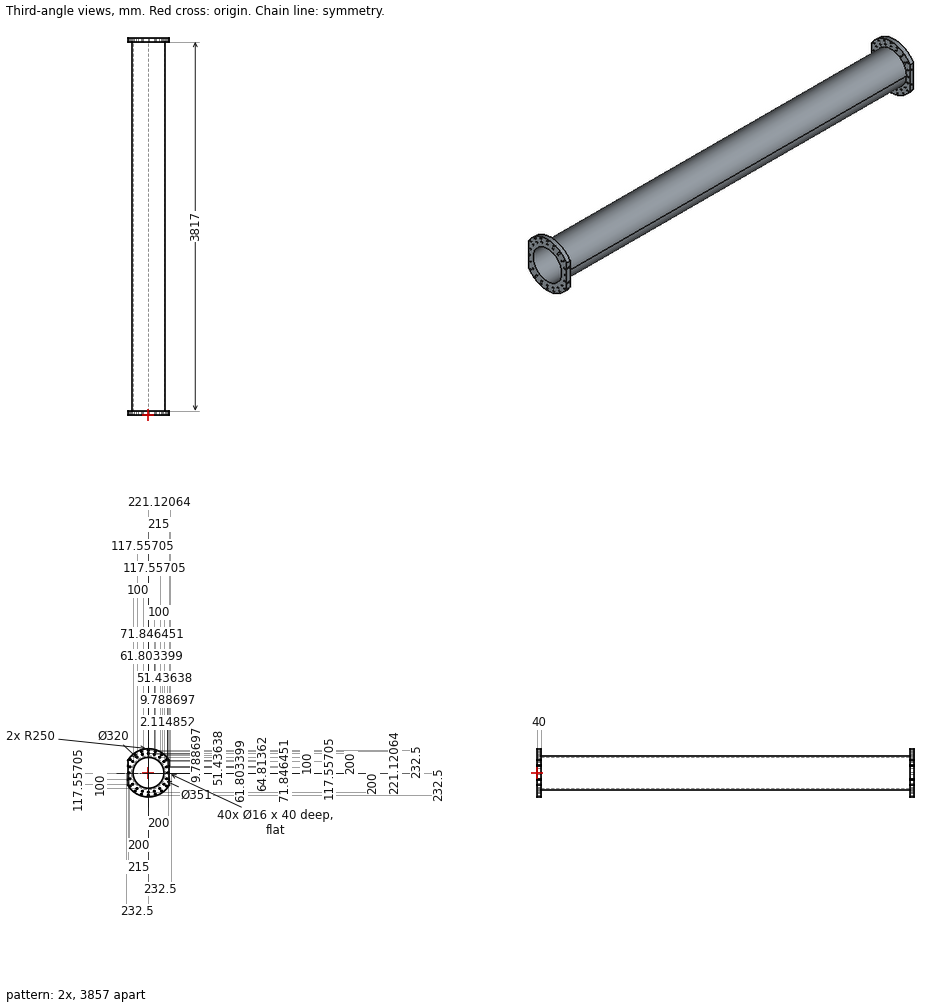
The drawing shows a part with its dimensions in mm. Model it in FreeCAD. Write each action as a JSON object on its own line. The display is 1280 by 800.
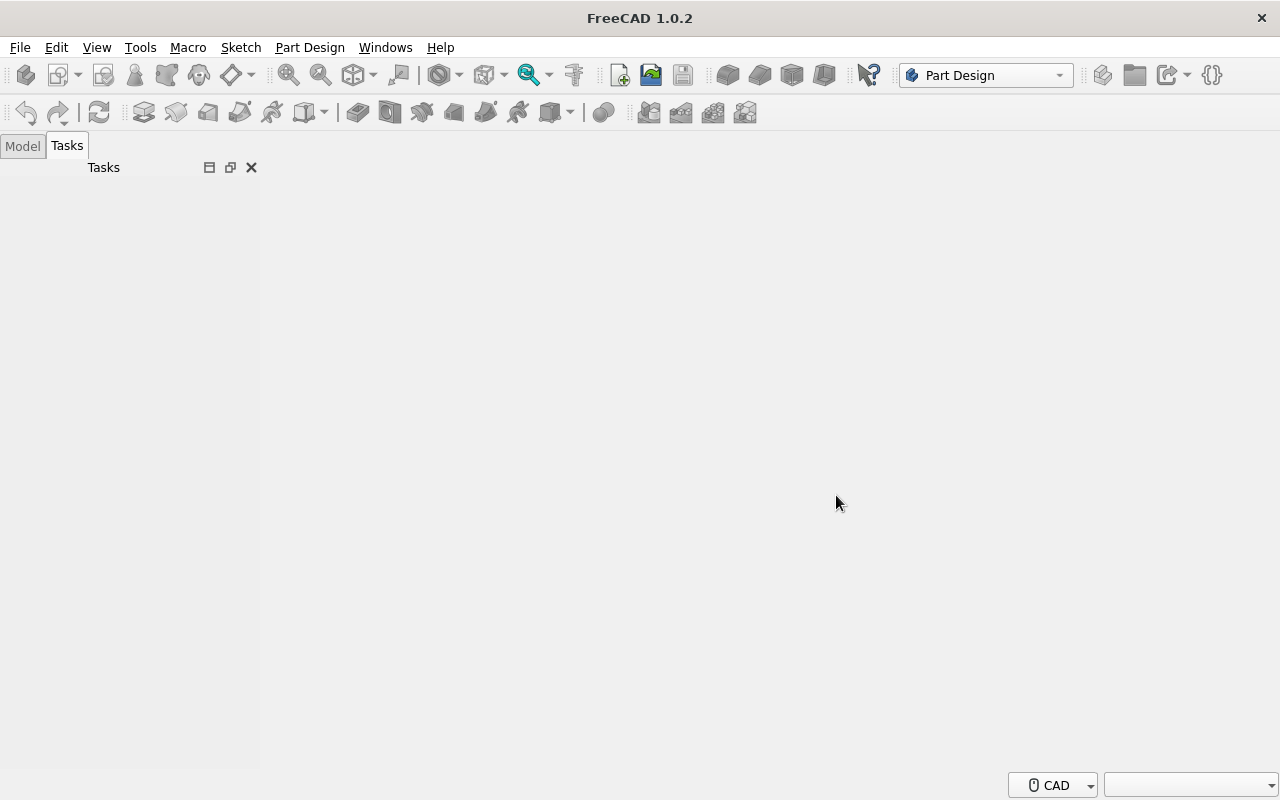
{"action": "left_click", "coordinate": [620, 76]}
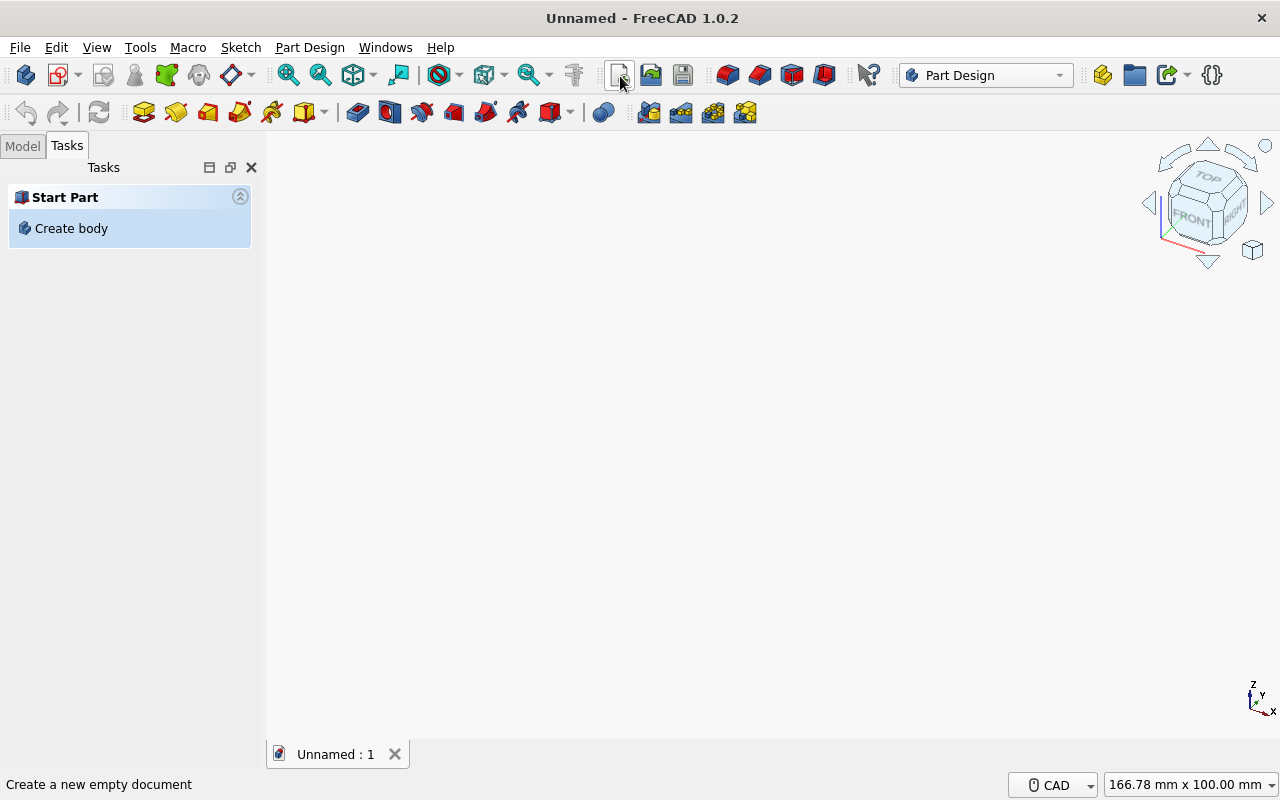
{"action": "left_click", "coordinate": [58, 76]}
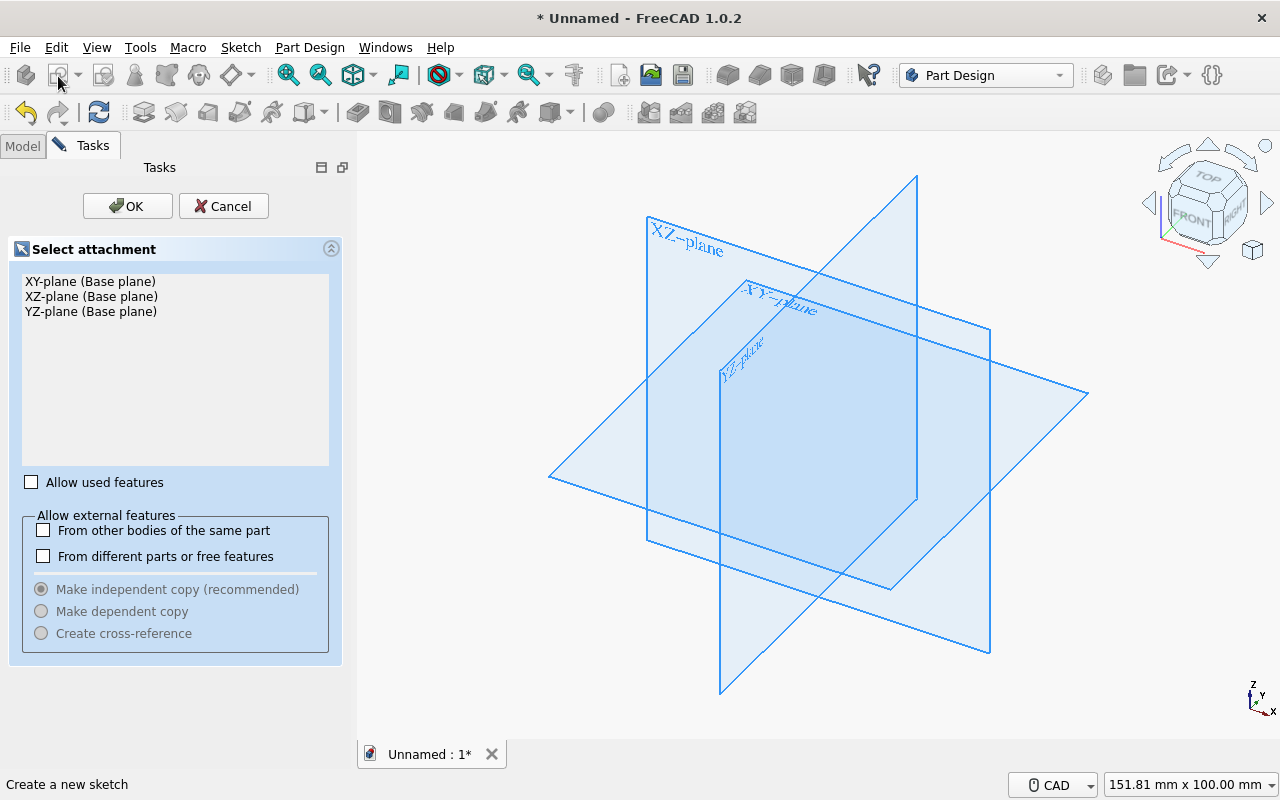
{"action": "left_click", "coordinate": [82, 296]}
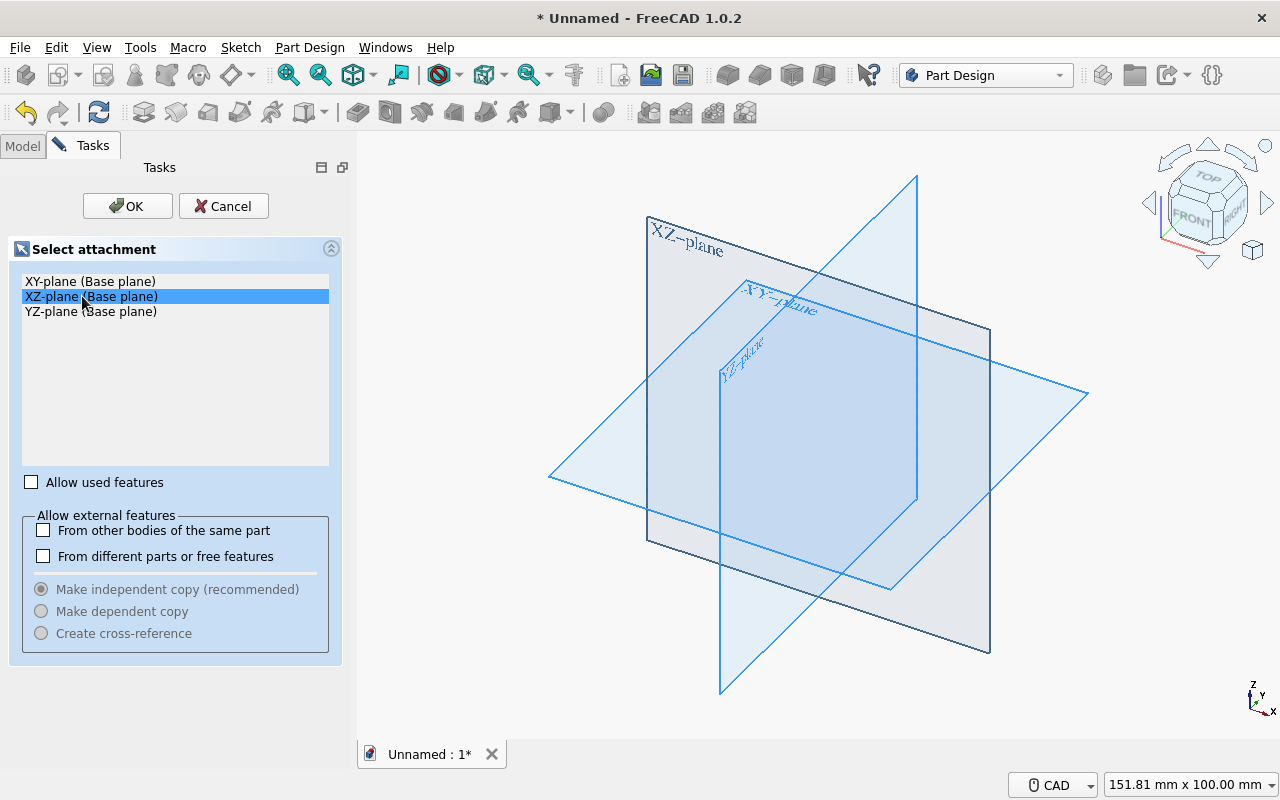
{"action": "left_click", "coordinate": [128, 206]}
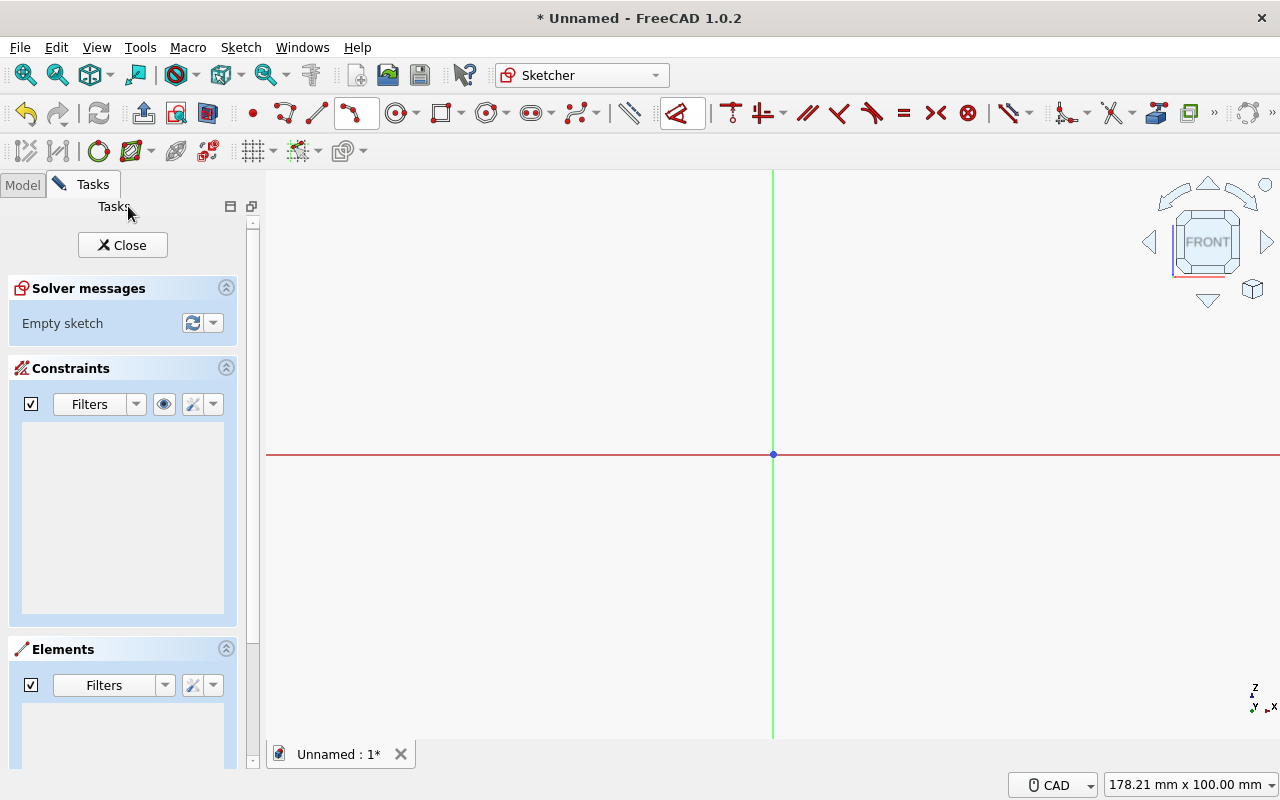
{"action": "scroll", "coordinate": [694, 454], "scroll_direction": "down", "scroll_amount": 10}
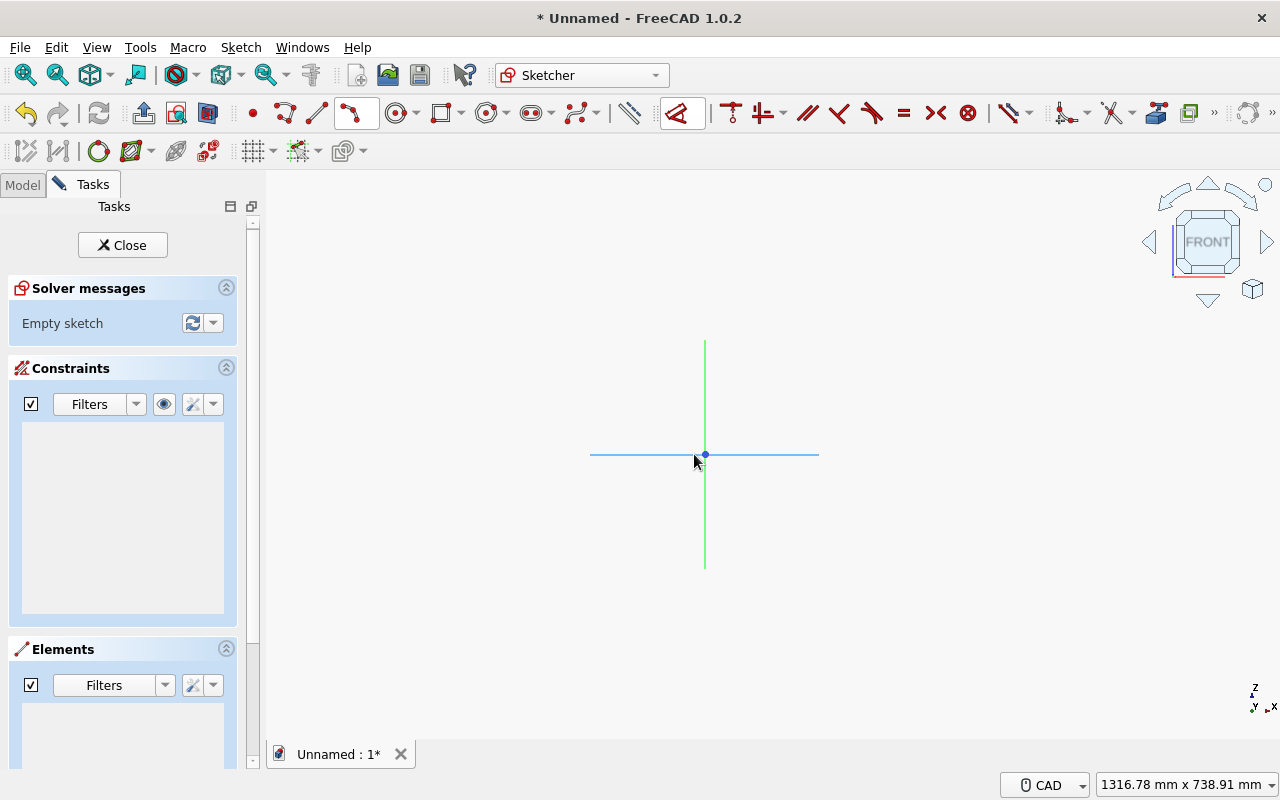
{"action": "left_click", "coordinate": [318, 114]}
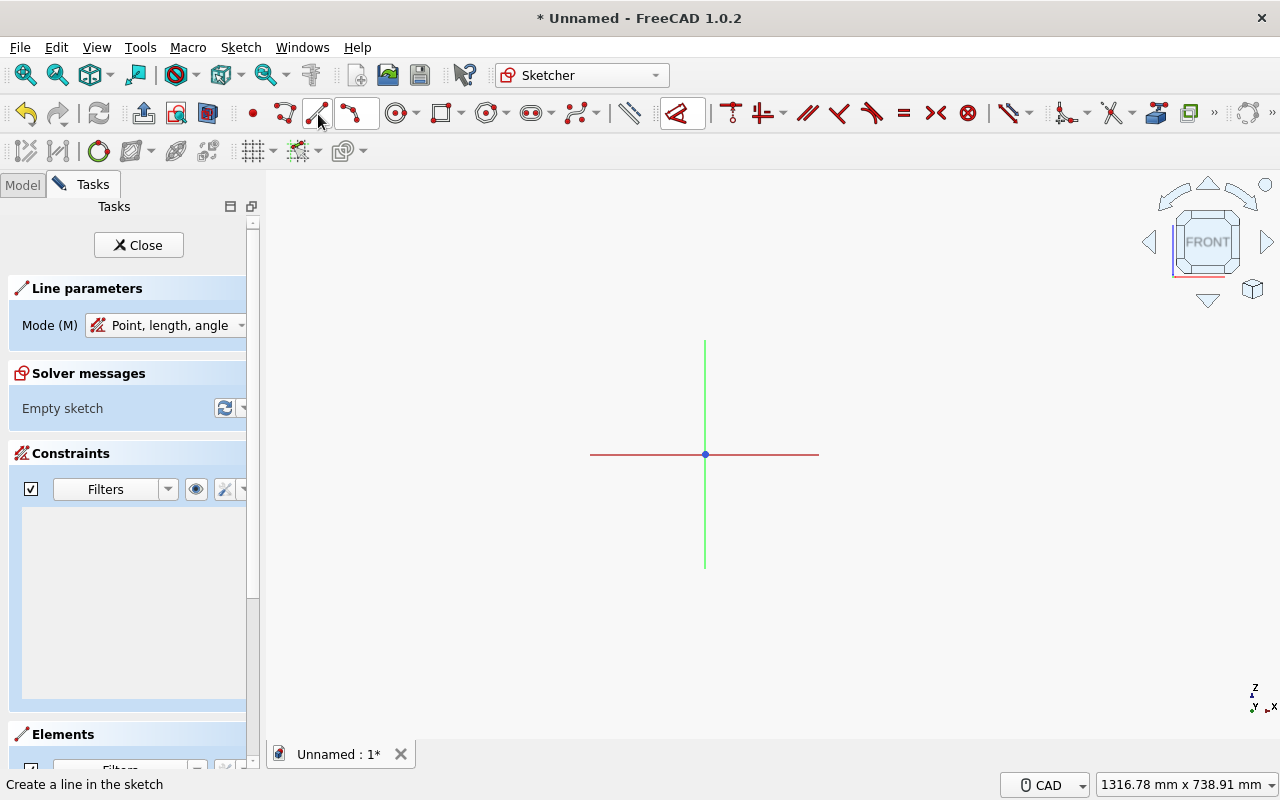
{"action": "left_click", "coordinate": [871, 356]}
{"action": "left_click", "coordinate": [871, 553]}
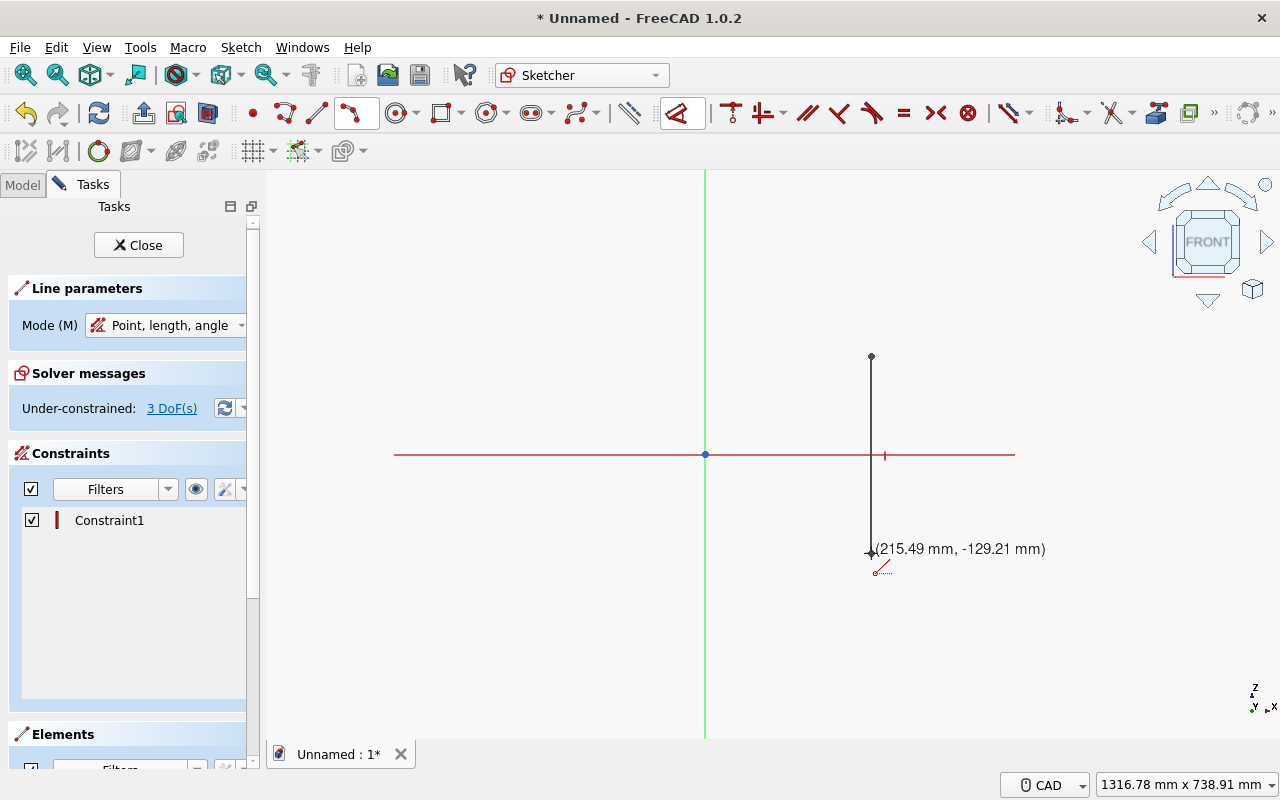
{"action": "left_click", "coordinate": [539, 553]}
{"action": "left_click", "coordinate": [539, 356]}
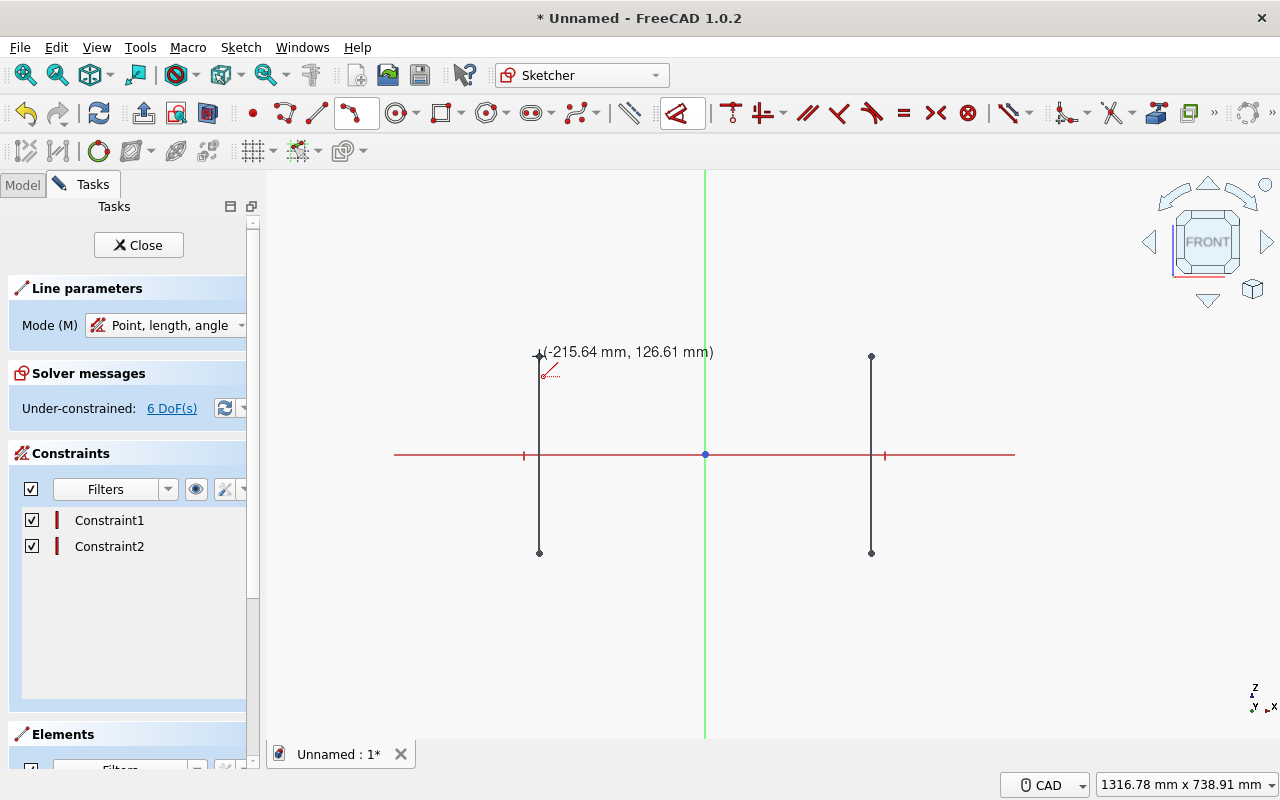
{"action": "key", "text": "g 3 a"}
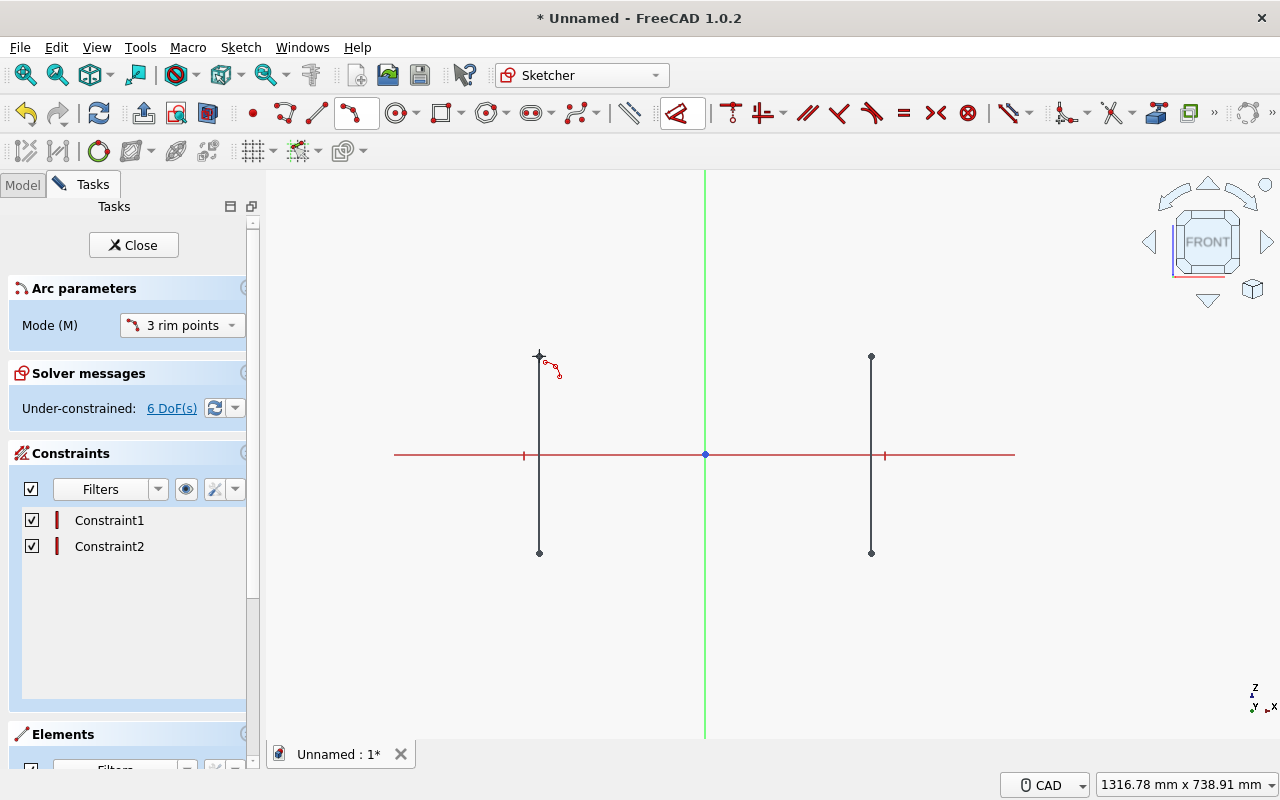
{"action": "left_click", "coordinate": [871, 554]}
{"action": "left_click", "coordinate": [539, 554]}
{"action": "left_click", "coordinate": [665, 643]}